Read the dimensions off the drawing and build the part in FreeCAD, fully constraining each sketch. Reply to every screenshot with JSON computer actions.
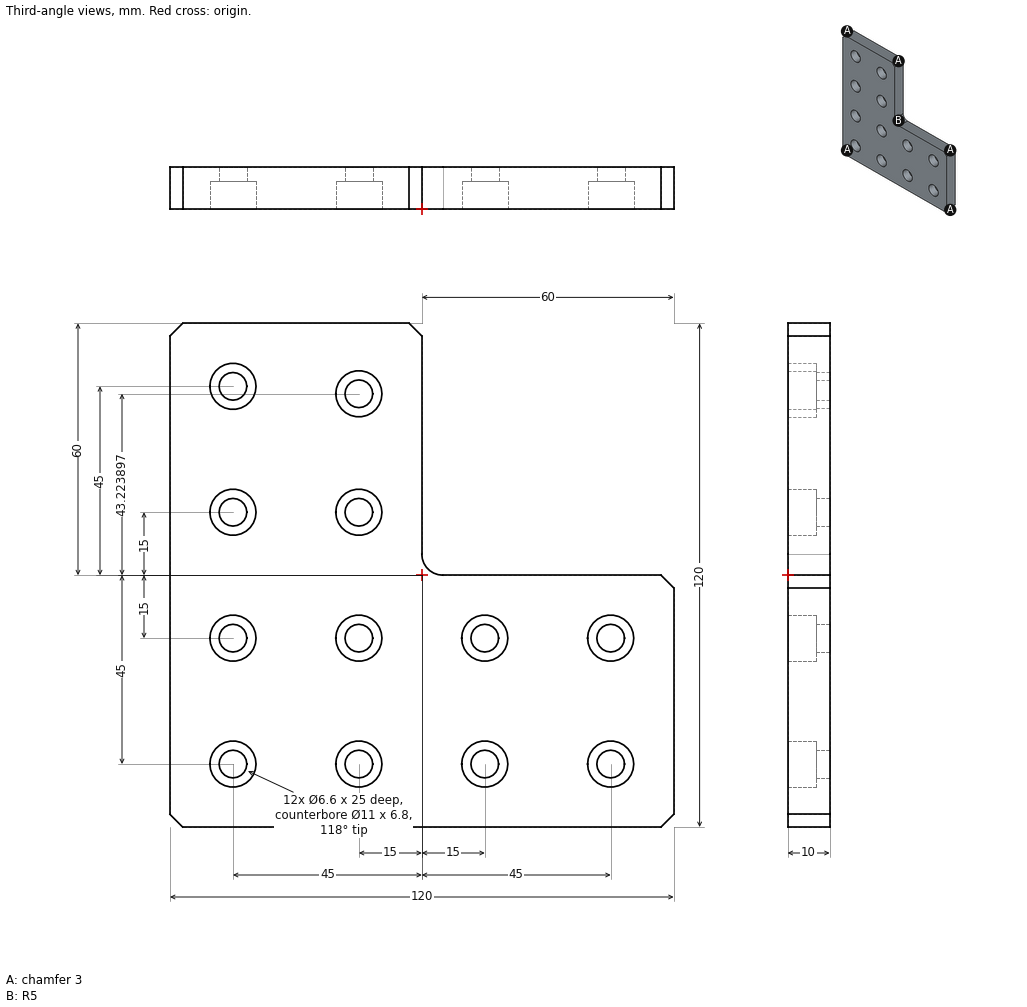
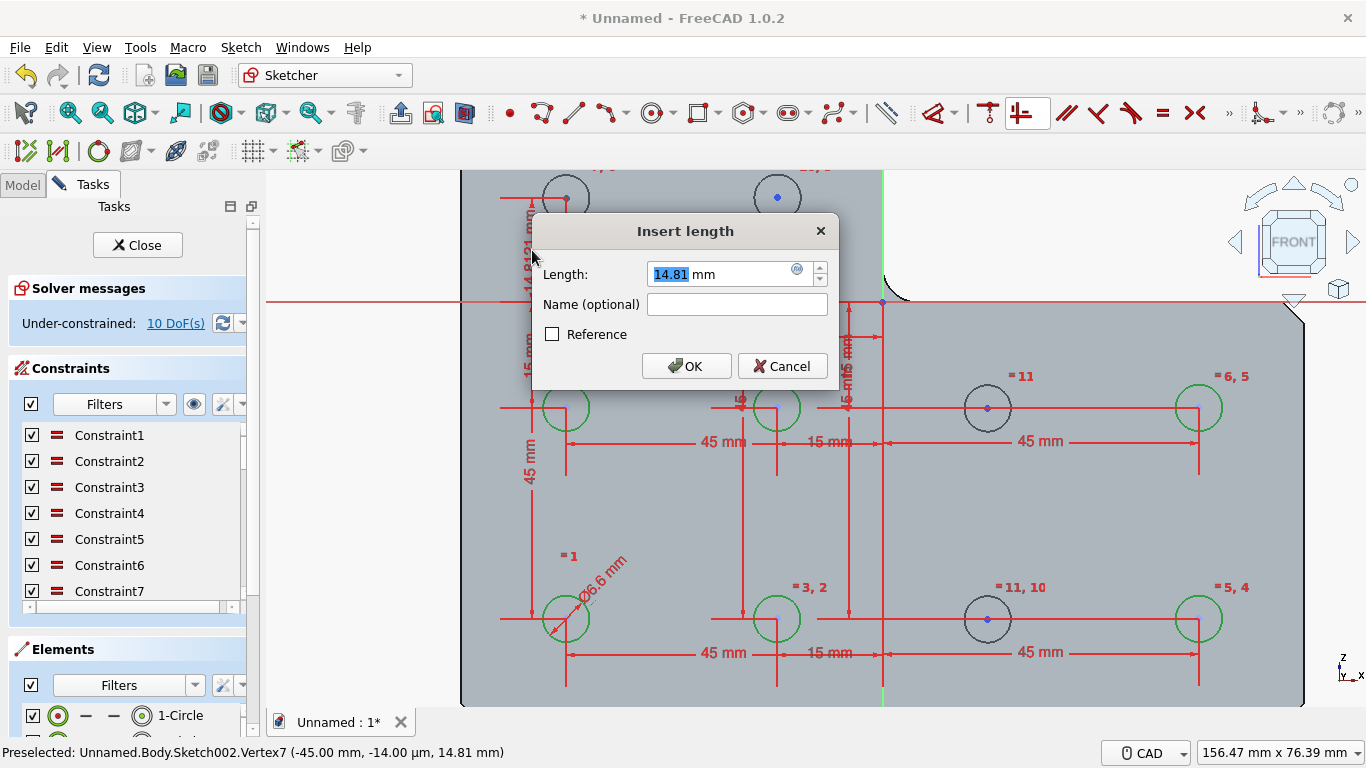
{"action": "type", "text": "15"}
{"action": "key", "text": "Return"}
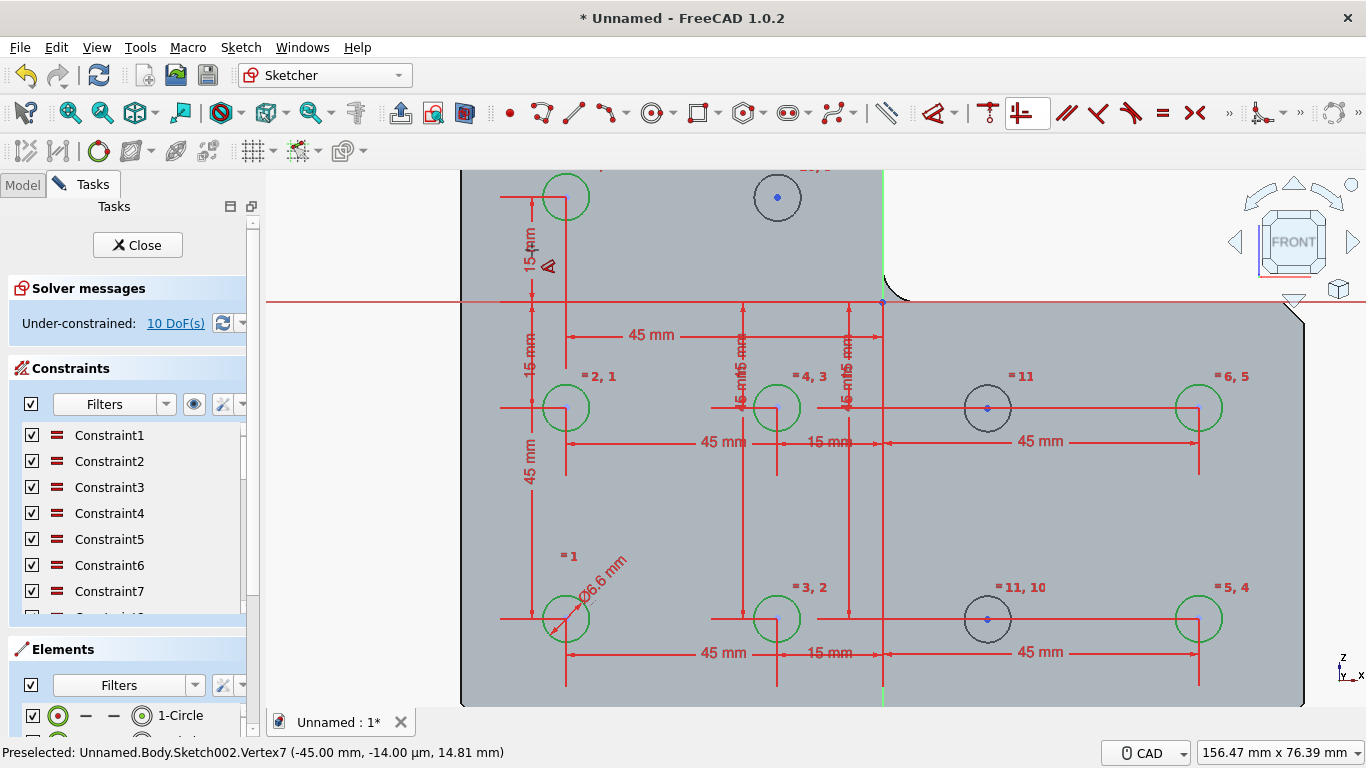
{"action": "scroll", "coordinate": [583, 604], "scroll_direction": "down", "scroll_amount": 3}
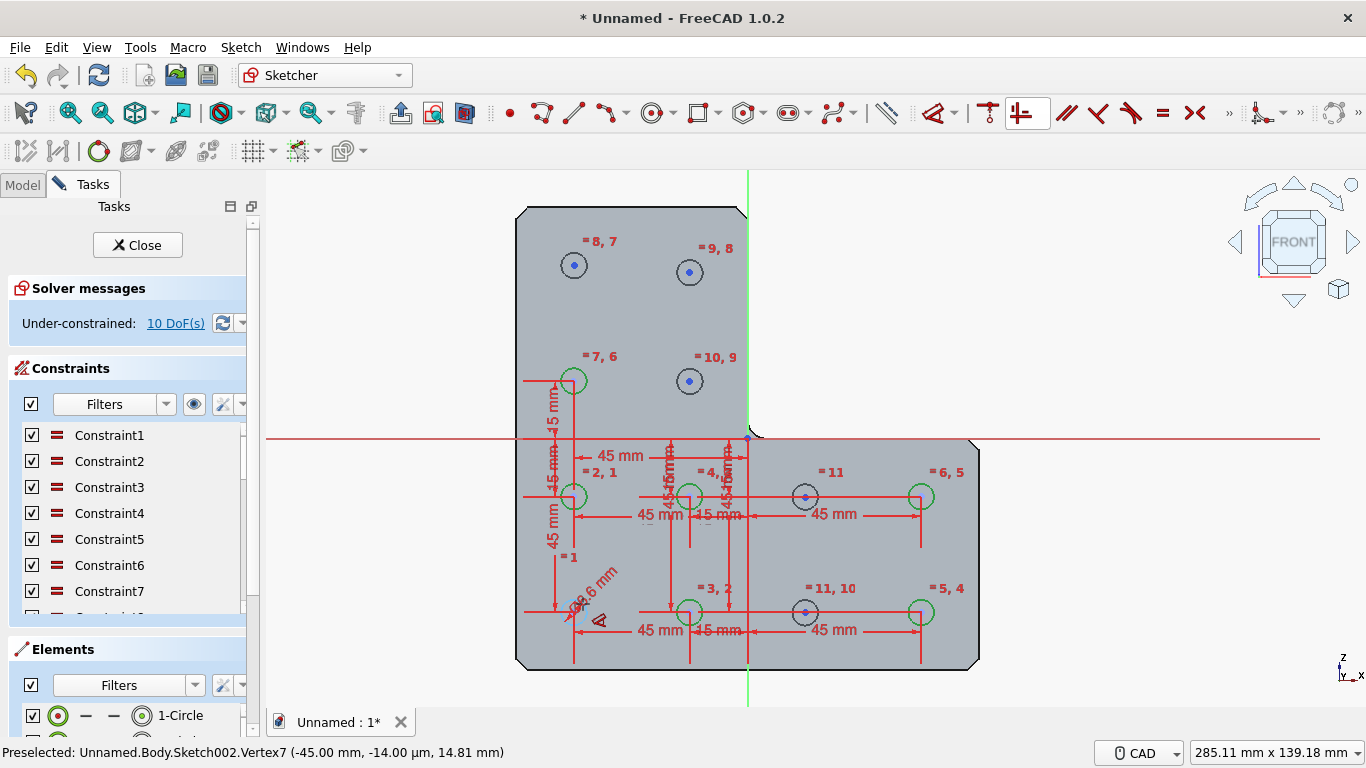
{"action": "left_click", "coordinate": [574, 266]}
{"action": "left_click", "coordinate": [661, 232]}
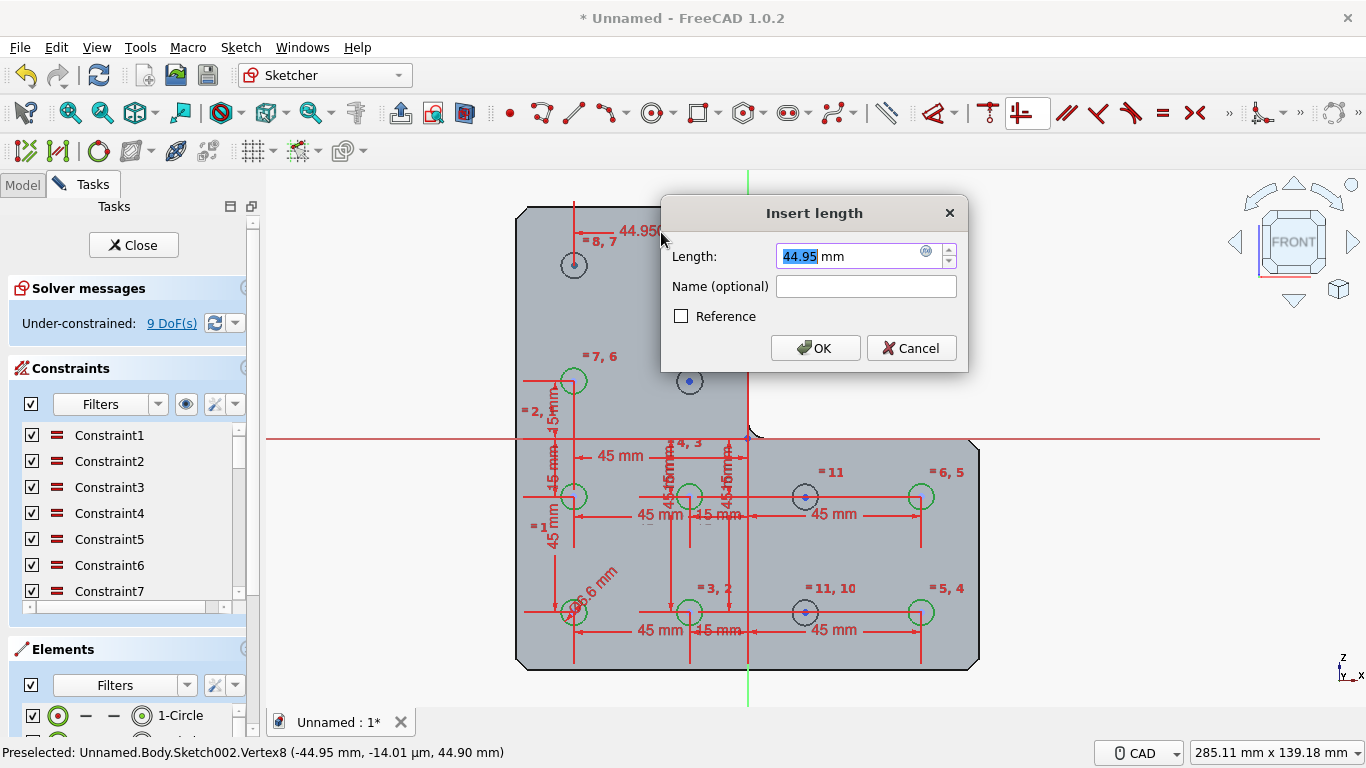
{"action": "type", "text": "45"}
{"action": "key", "text": "Return"}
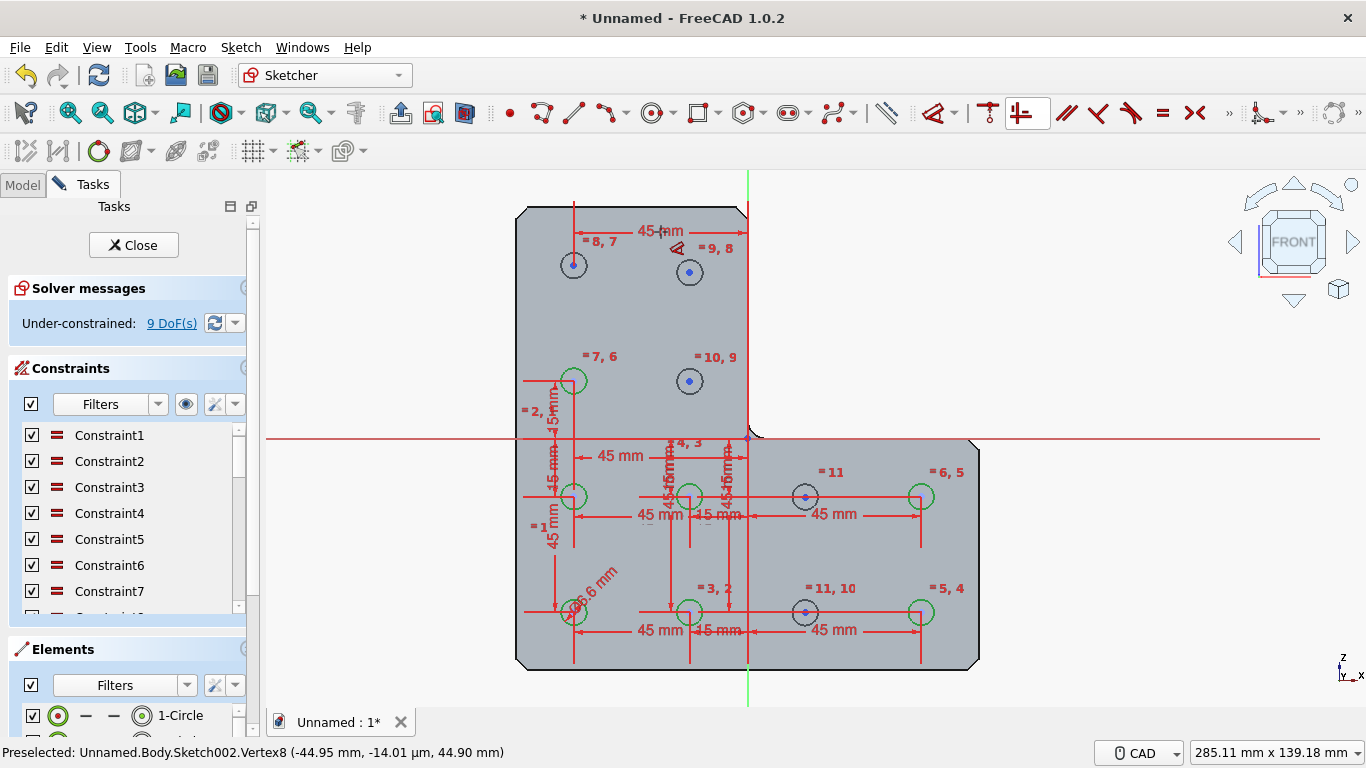
{"action": "left_click", "coordinate": [574, 266]}
{"action": "left_click", "coordinate": [540, 352]}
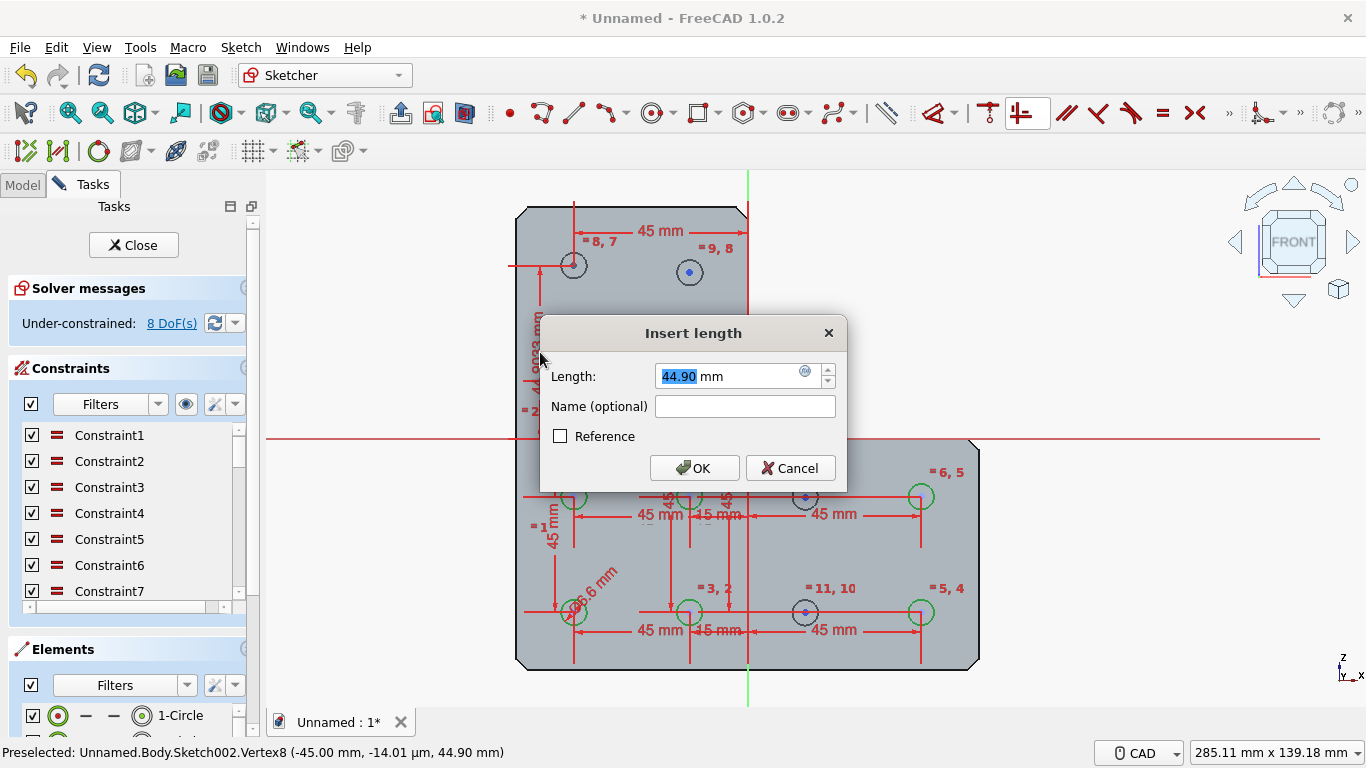
{"action": "type", "text": "45"}
{"action": "key", "text": "Return"}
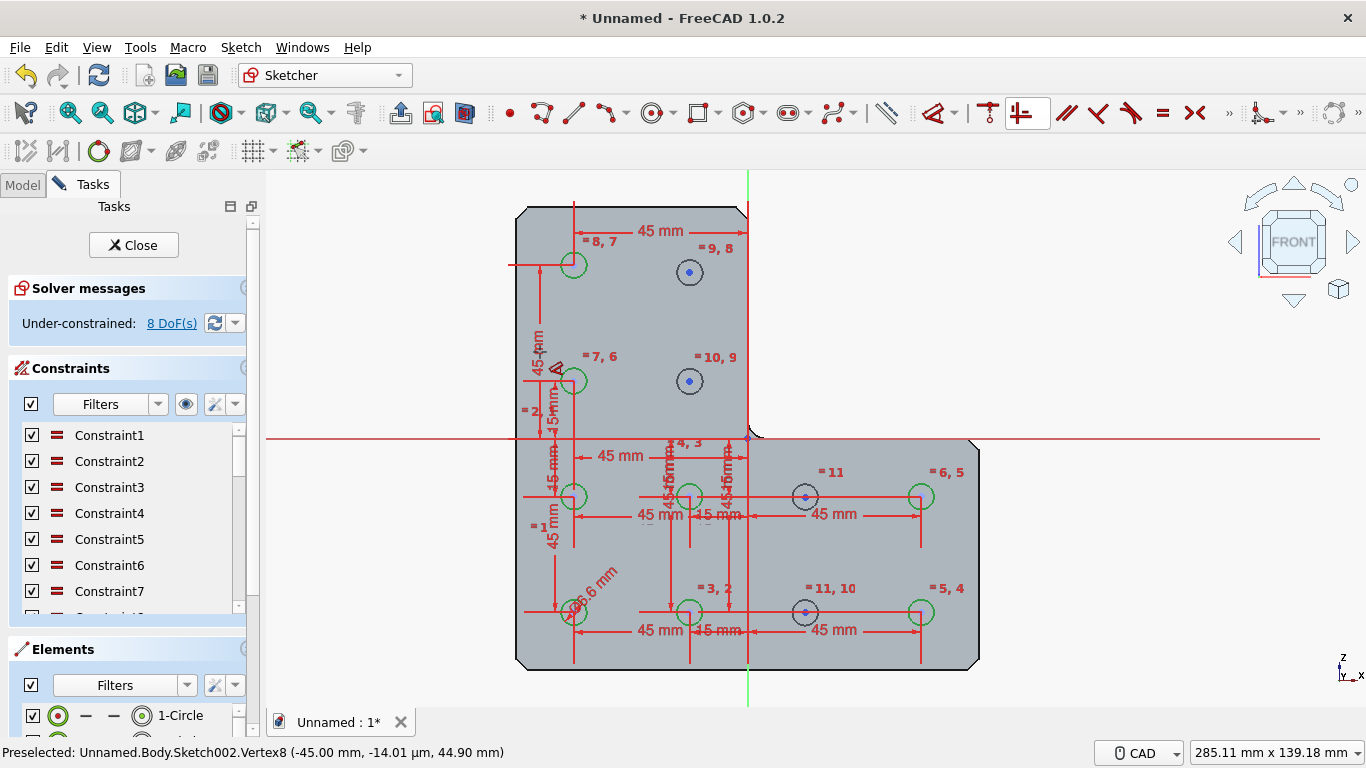
{"action": "left_click", "coordinate": [690, 273]}
{"action": "left_click", "coordinate": [732, 239]}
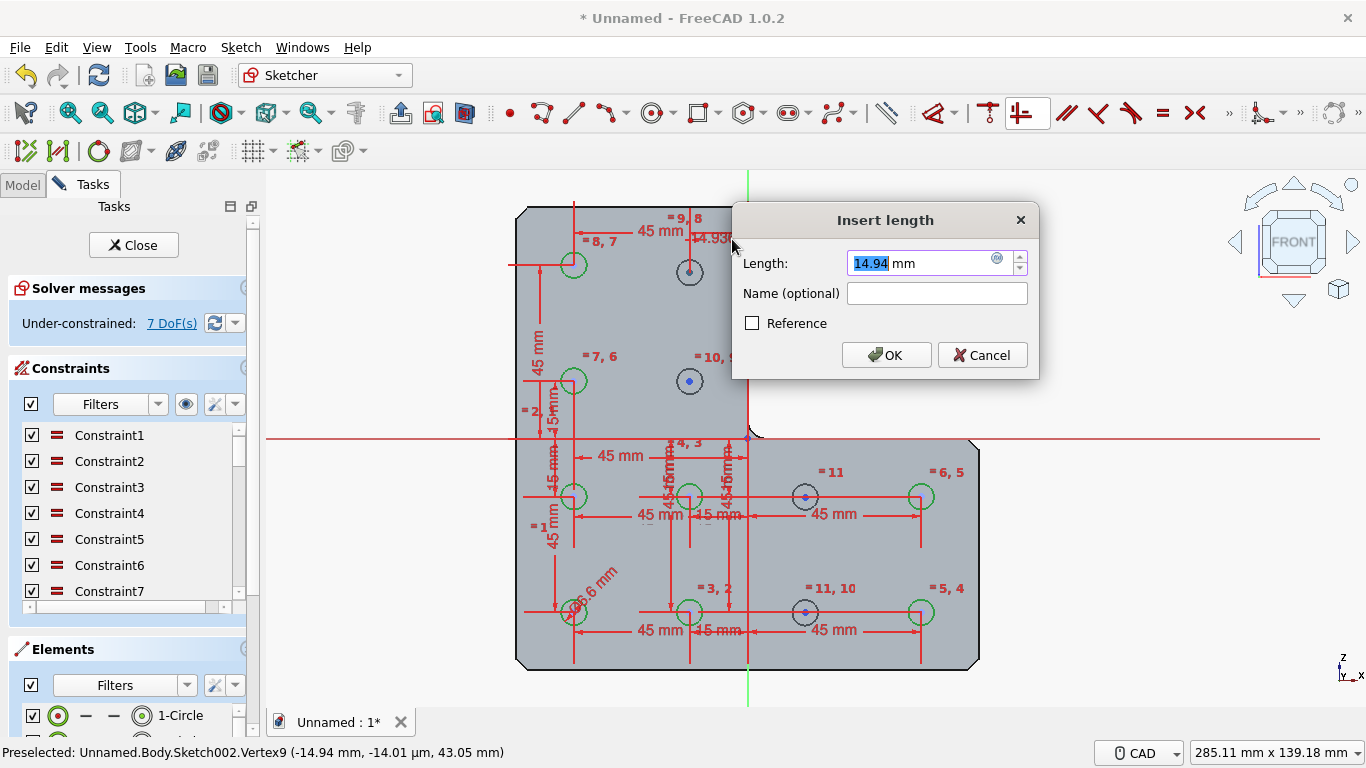
{"action": "type", "text": "15"}
{"action": "key", "text": "Return"}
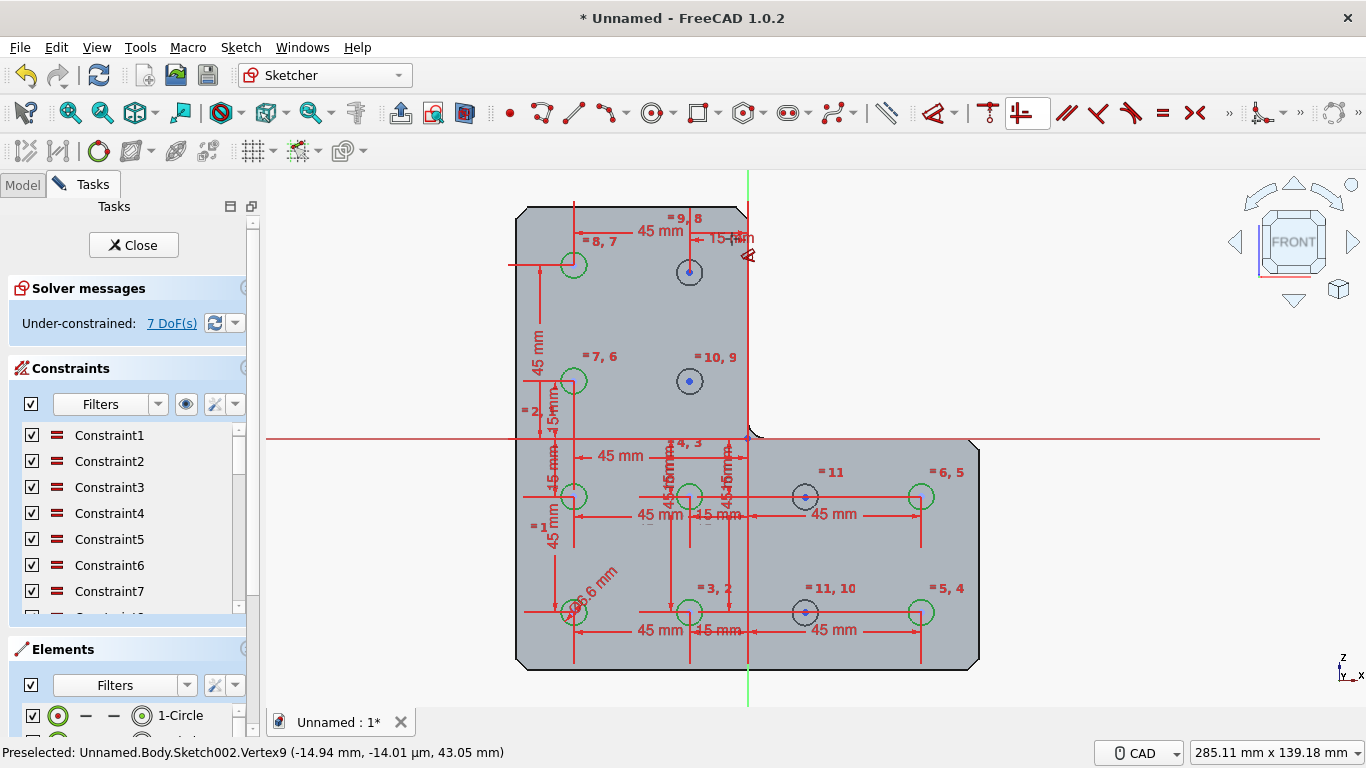
{"action": "left_click", "coordinate": [690, 381]}
{"action": "left_click", "coordinate": [719, 347]}